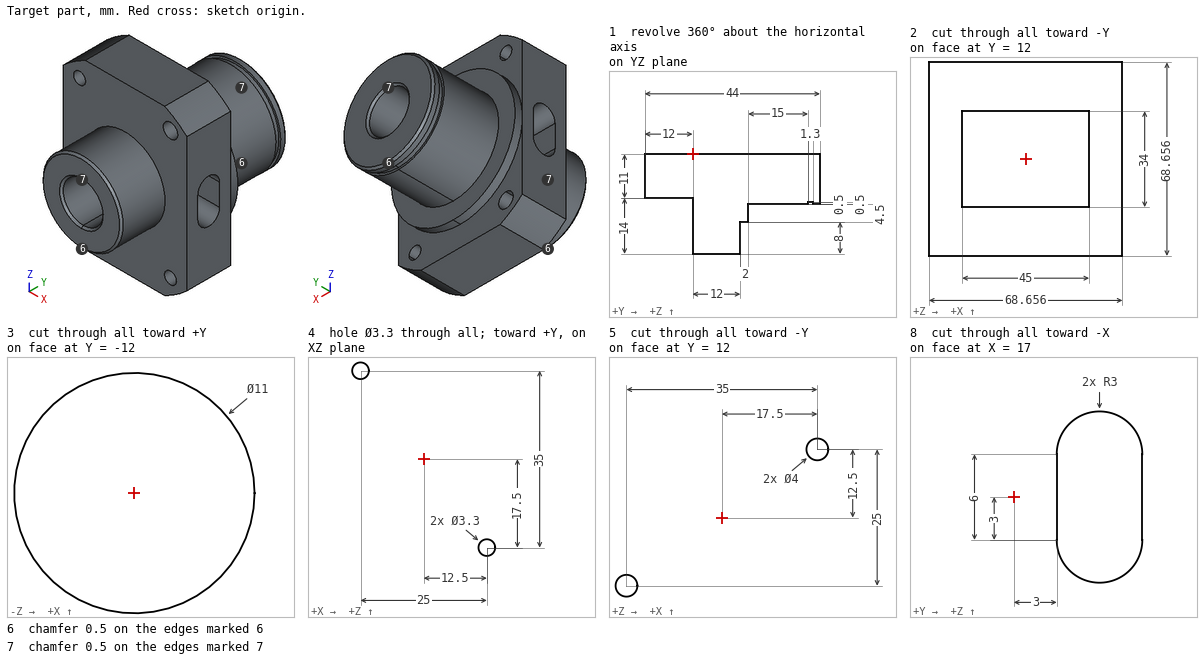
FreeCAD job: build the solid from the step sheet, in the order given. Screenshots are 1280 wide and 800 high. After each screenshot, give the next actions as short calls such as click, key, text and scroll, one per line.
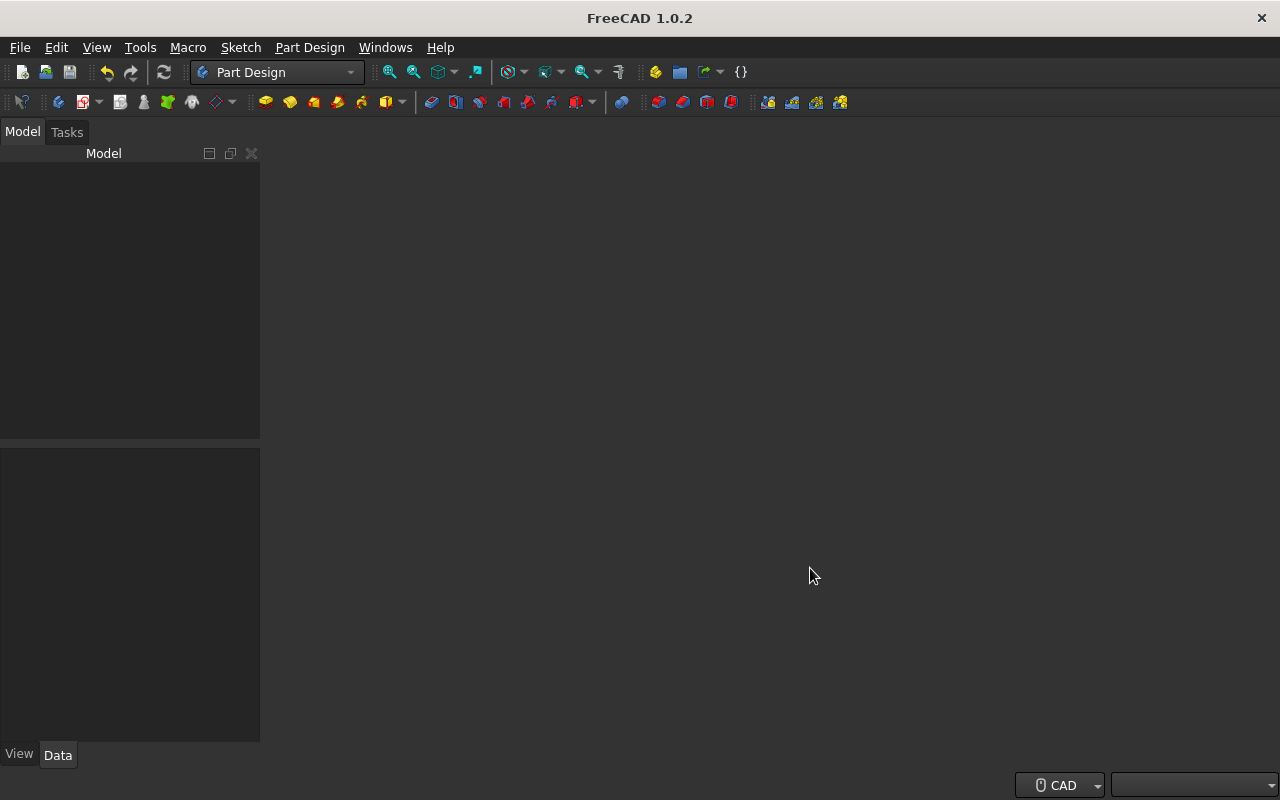
key(ctrl+n)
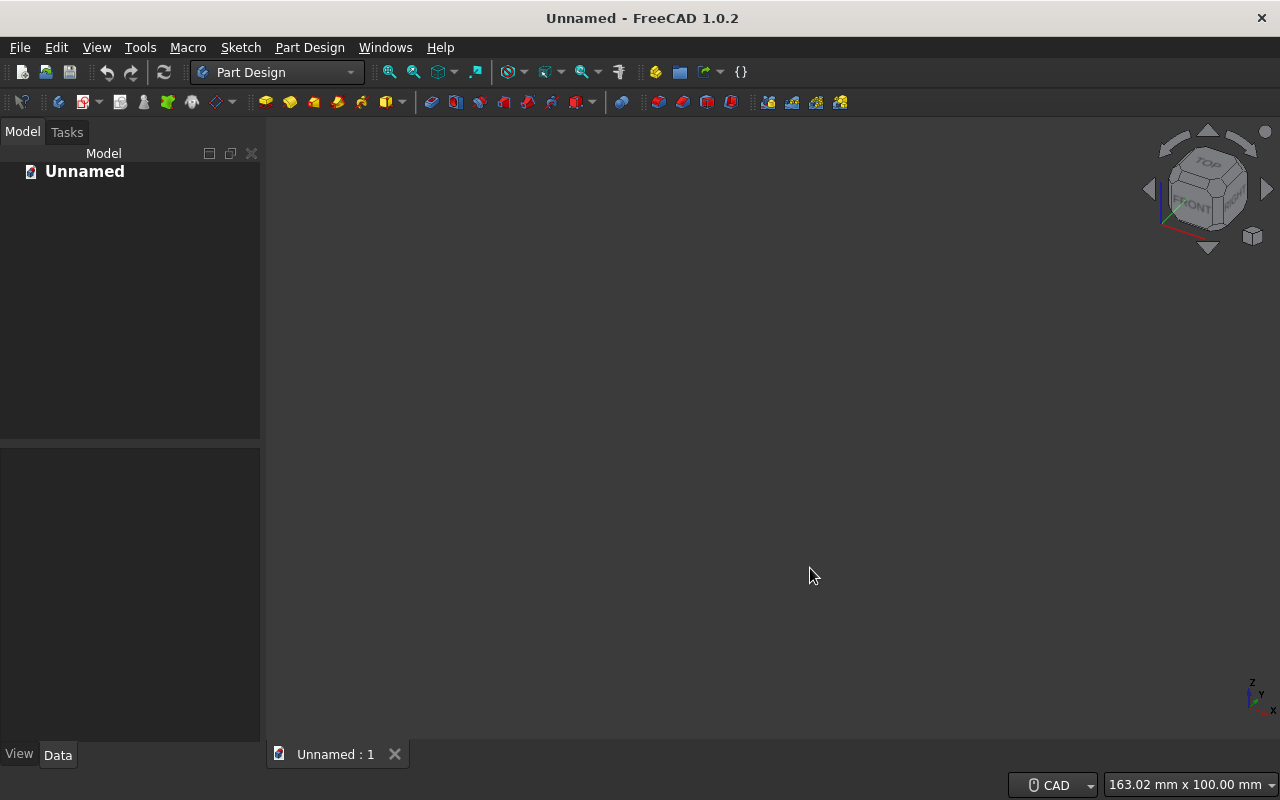
click(84, 102)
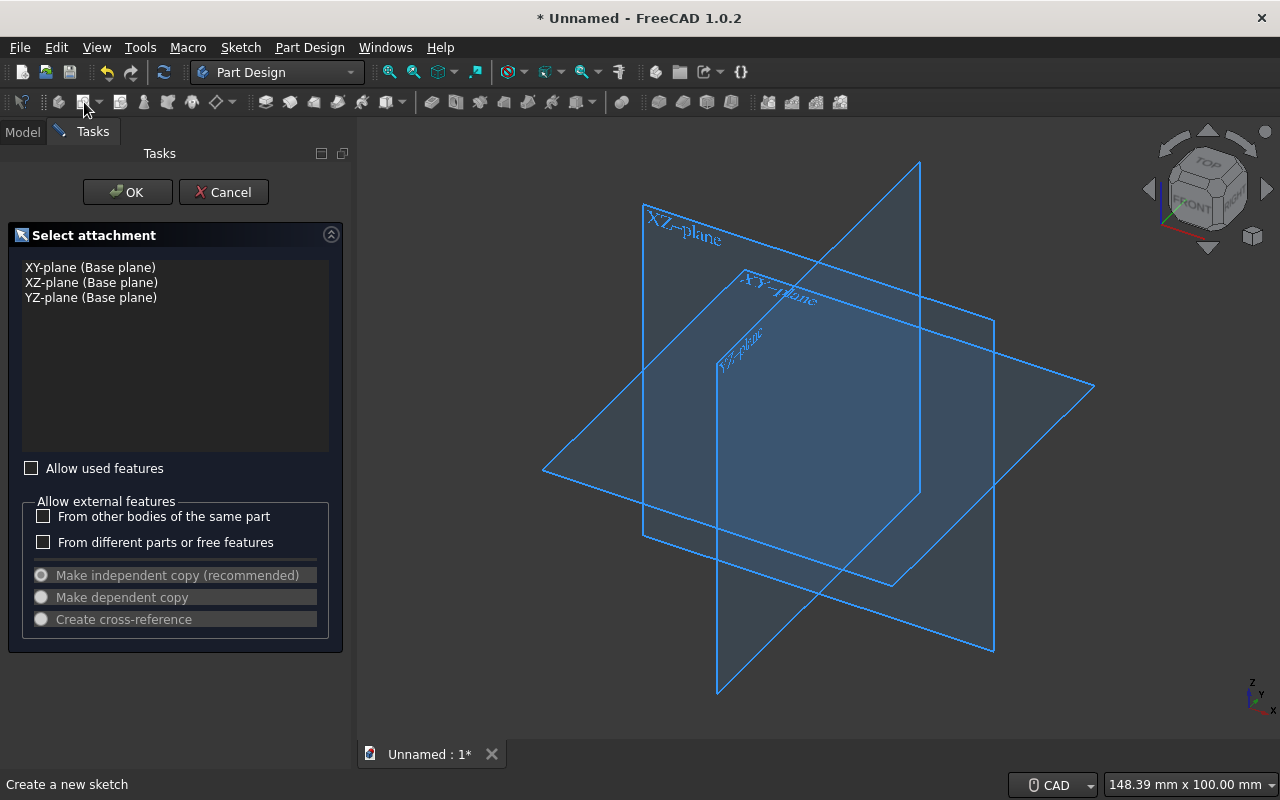
click(82, 298)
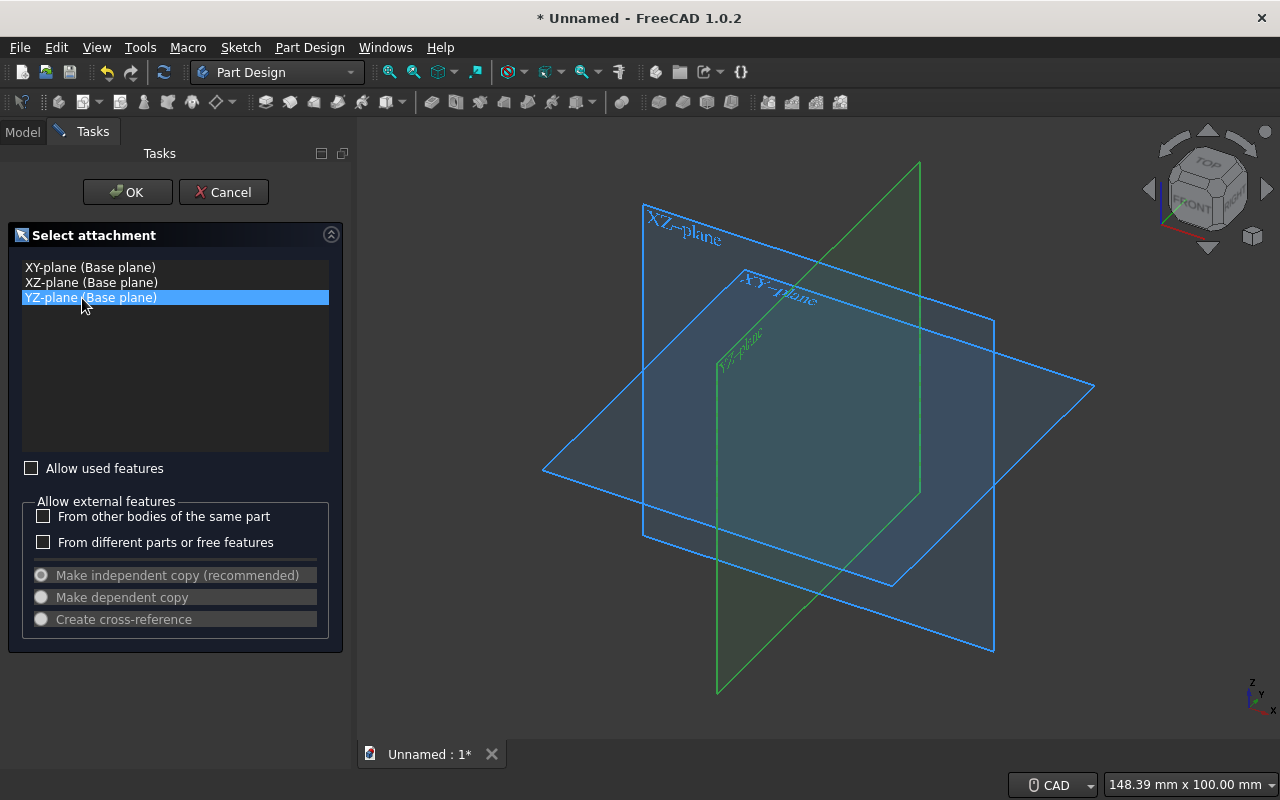
click(128, 192)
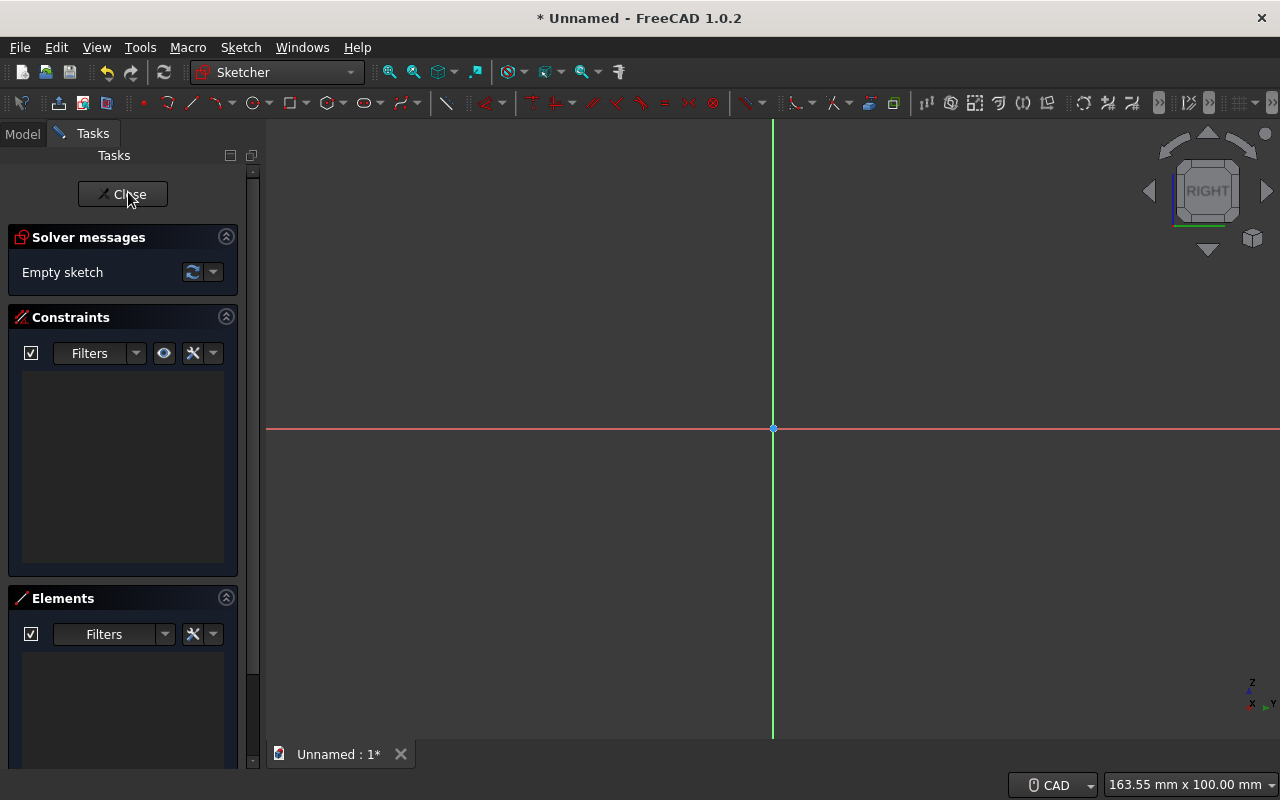
scroll(941, 570, up, 4)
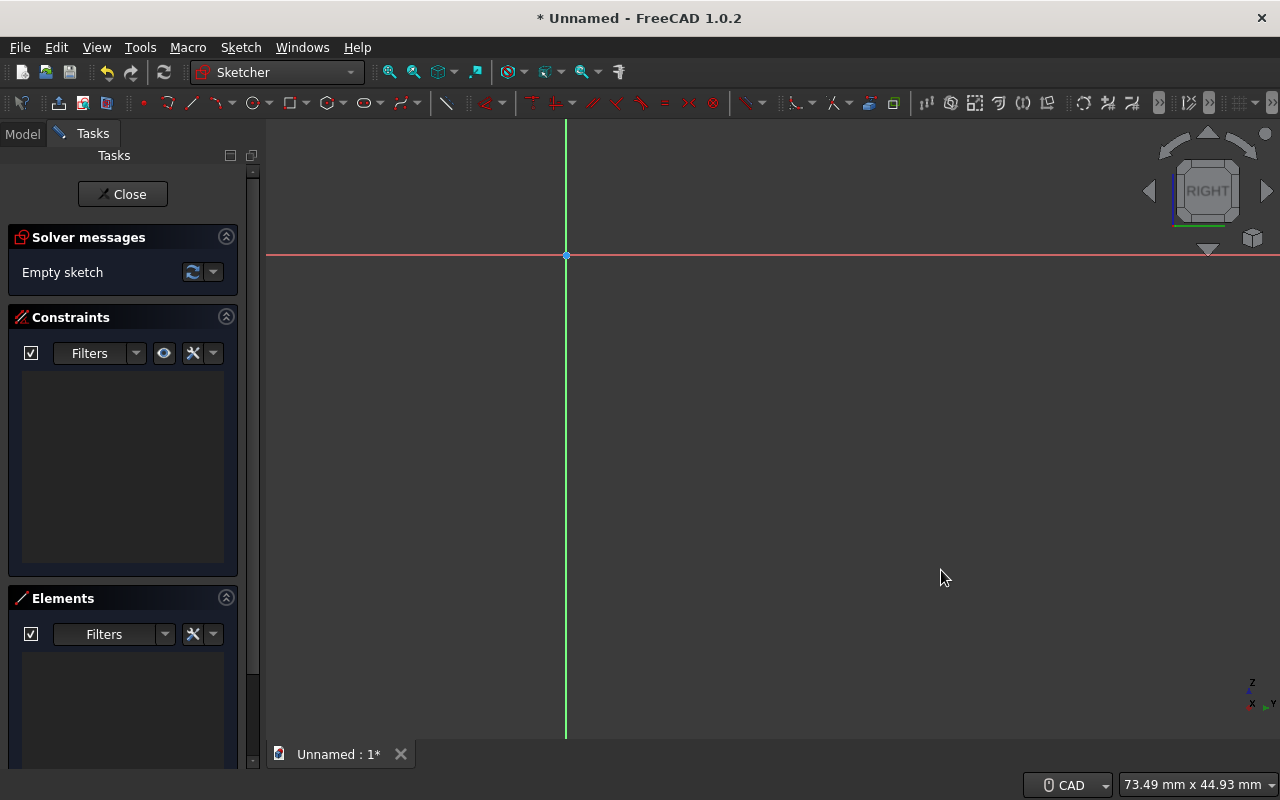
click(168, 104)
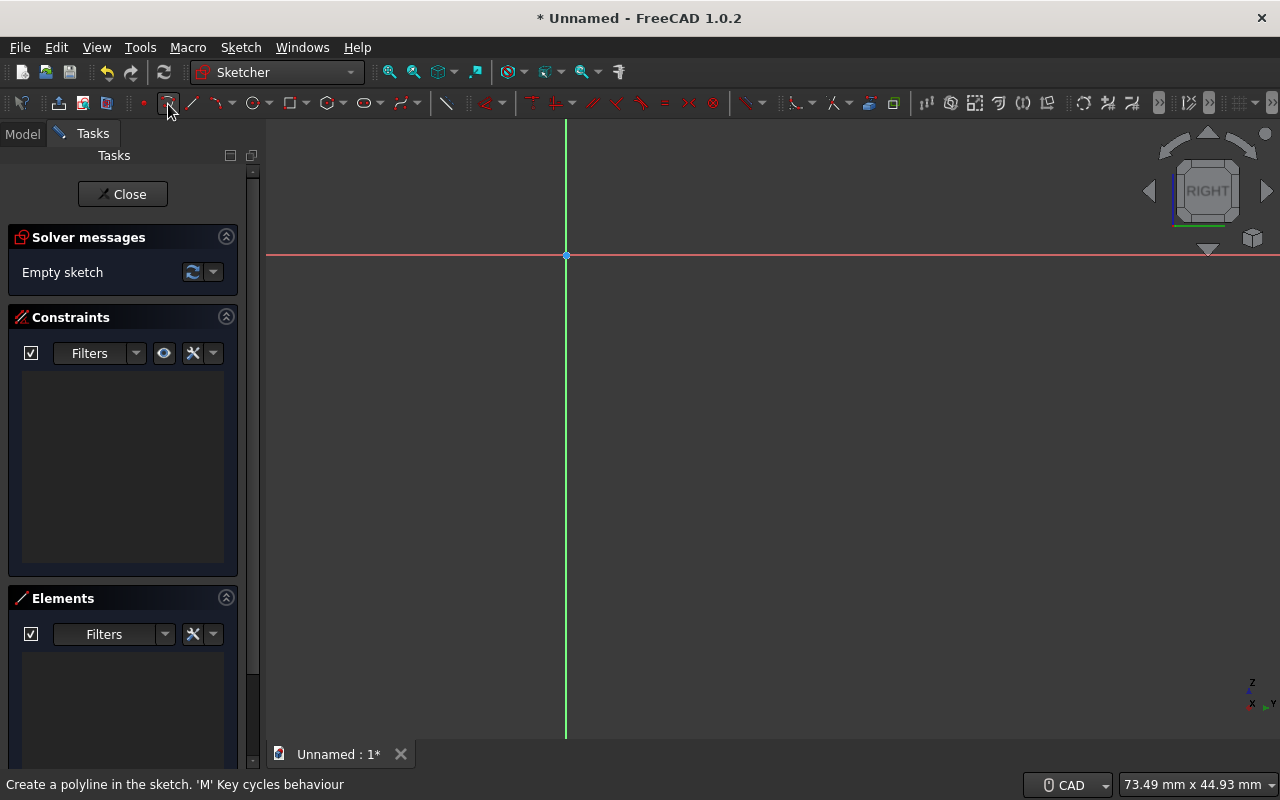
click(566, 407)
click(575, 600)
click(732, 600)
click(732, 490)
click(759, 490)
click(759, 428)
click(966, 428)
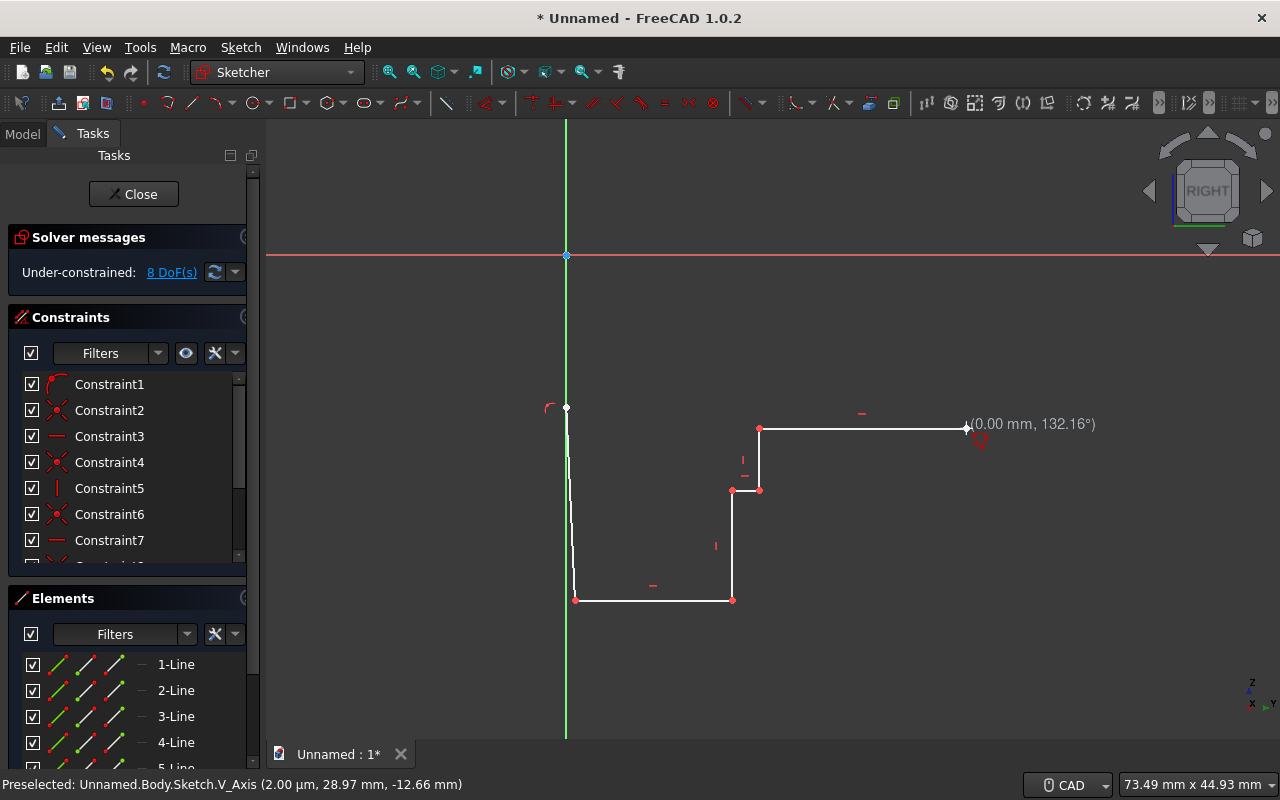
scroll(966, 421, up, 5)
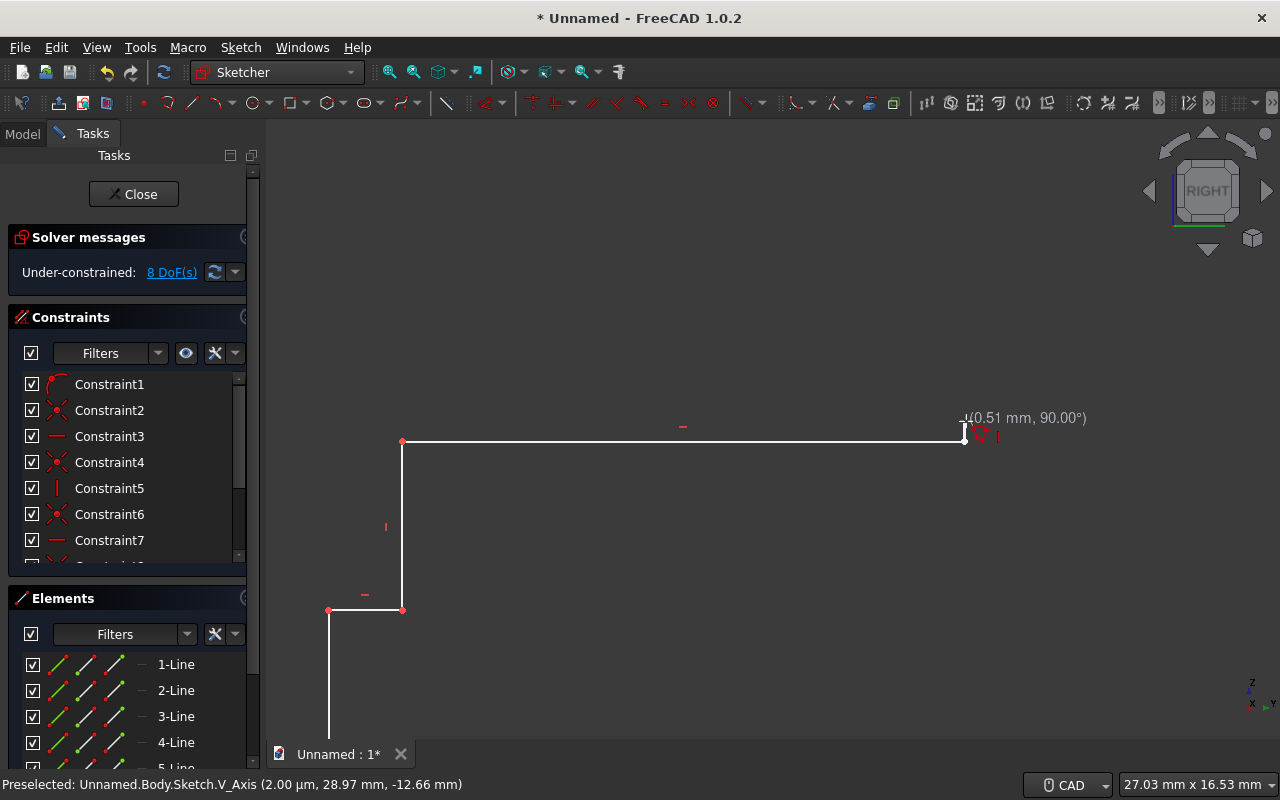
click(965, 420)
click(1015, 420)
click(1015, 439)
click(1079, 439)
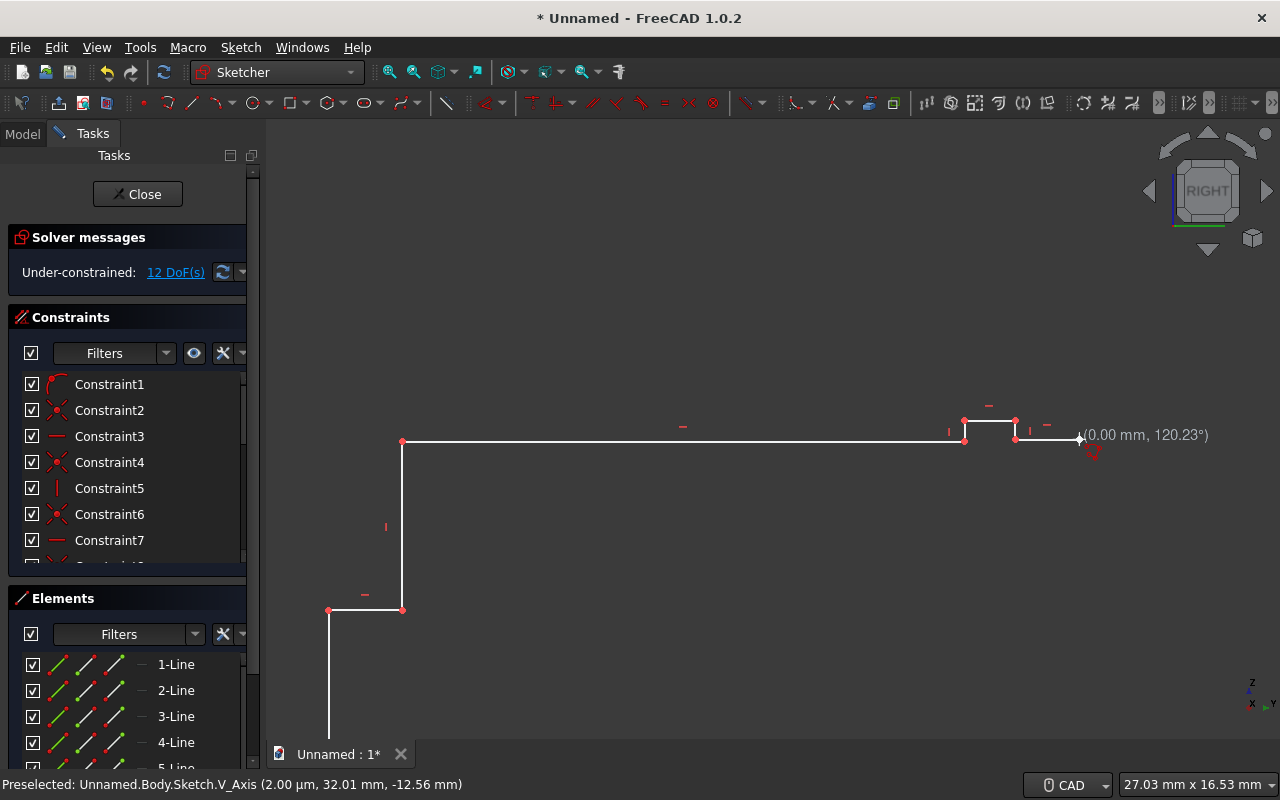
scroll(967, 423, down, 5)